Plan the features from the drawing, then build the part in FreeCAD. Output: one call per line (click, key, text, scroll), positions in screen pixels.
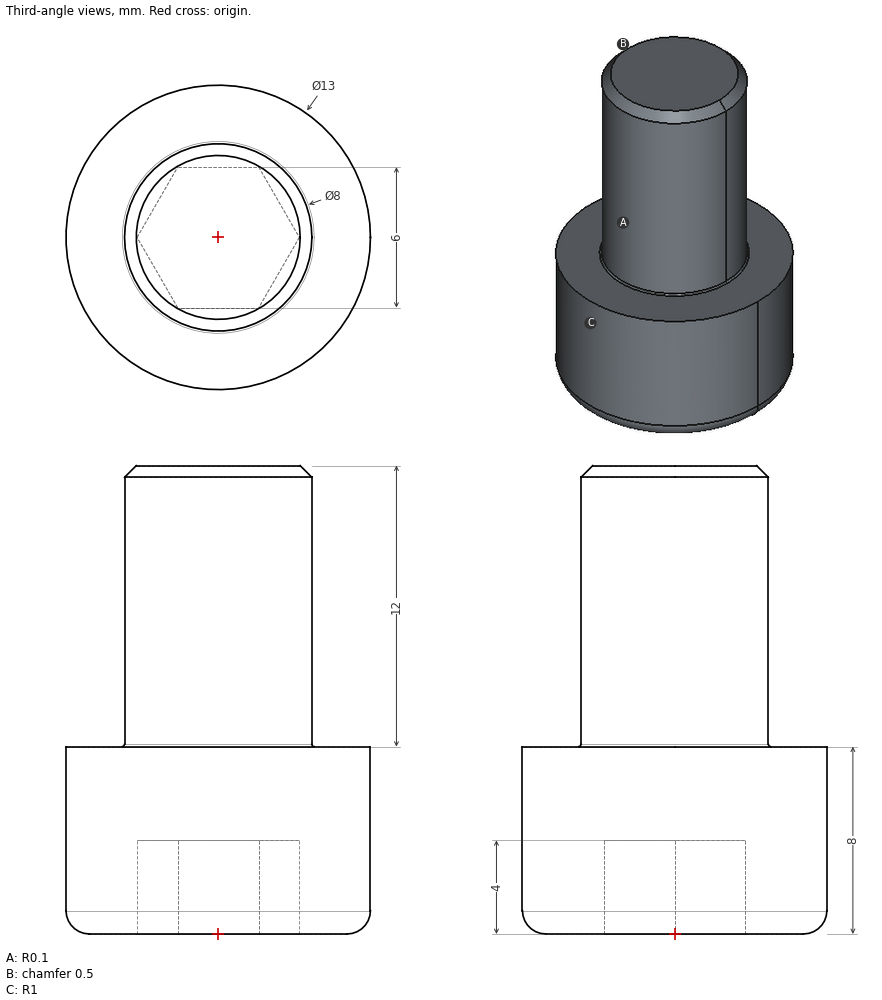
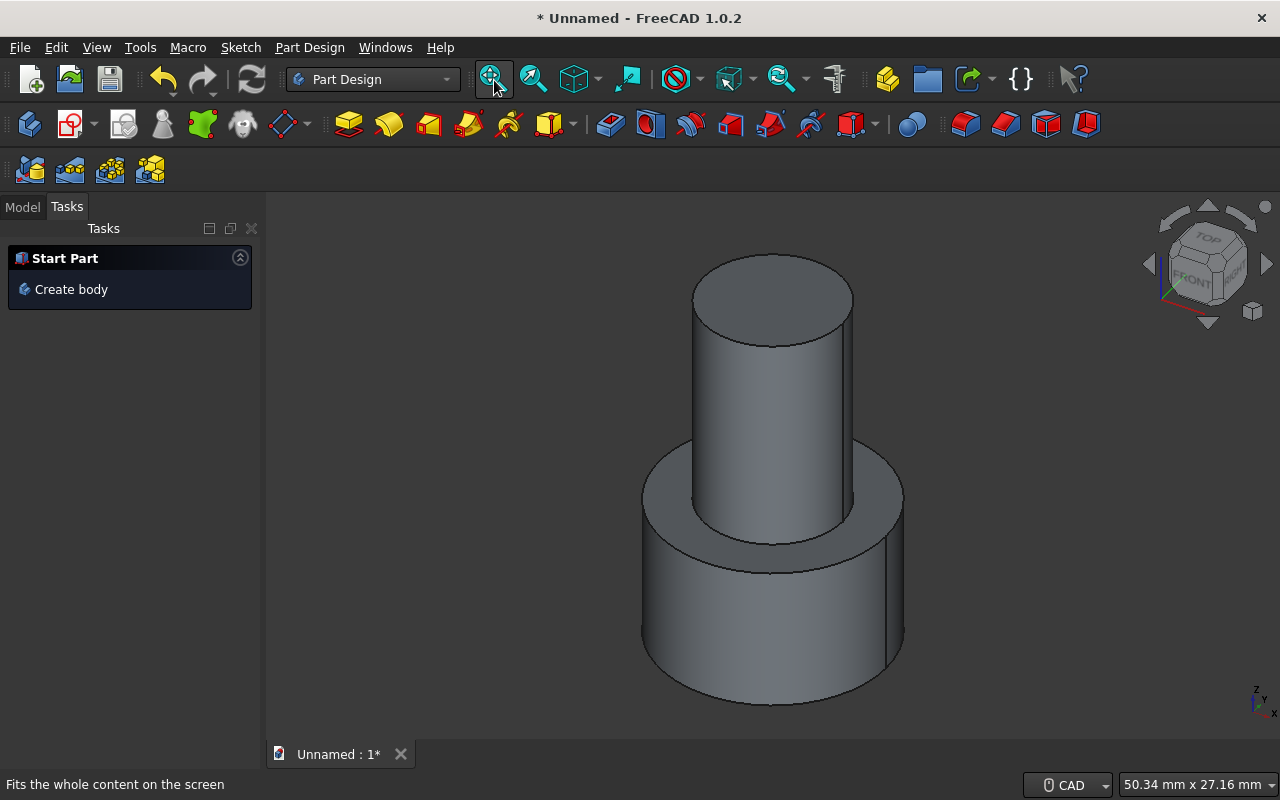
click(70, 124)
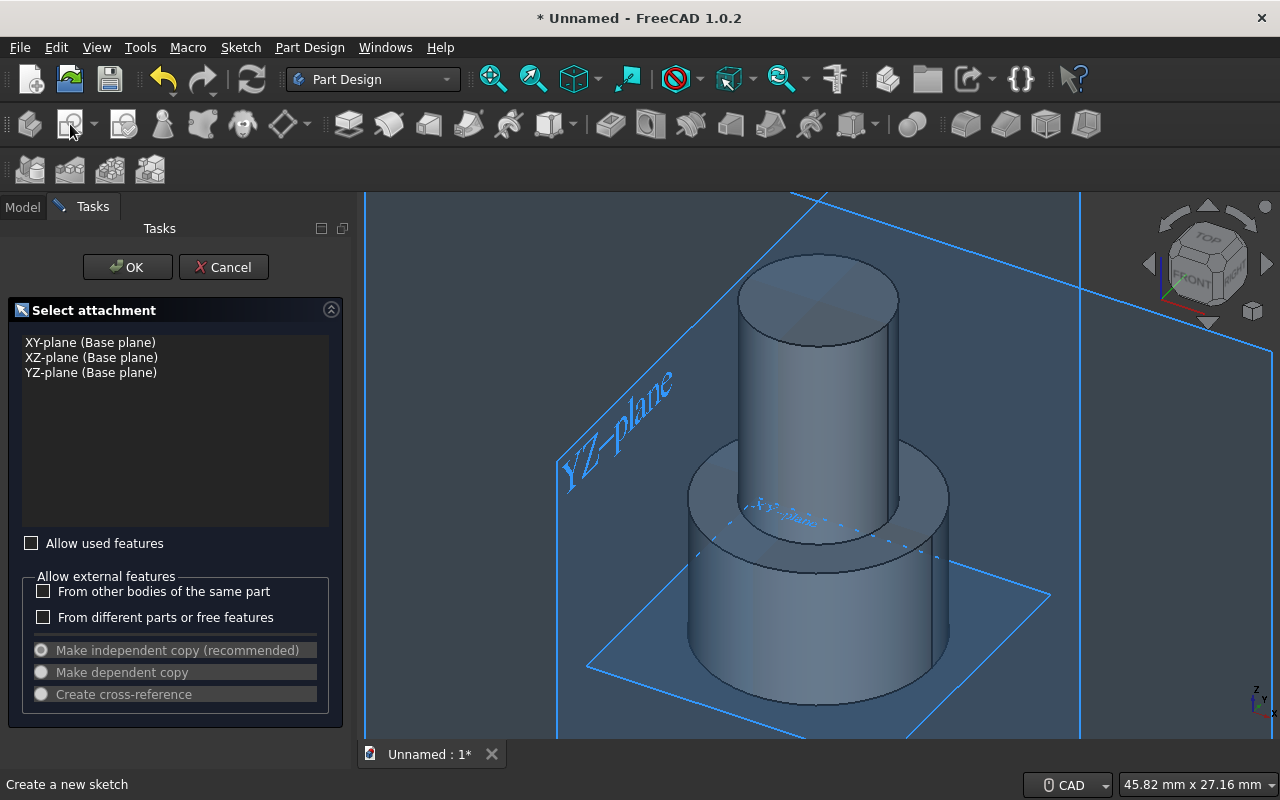
click(82, 342)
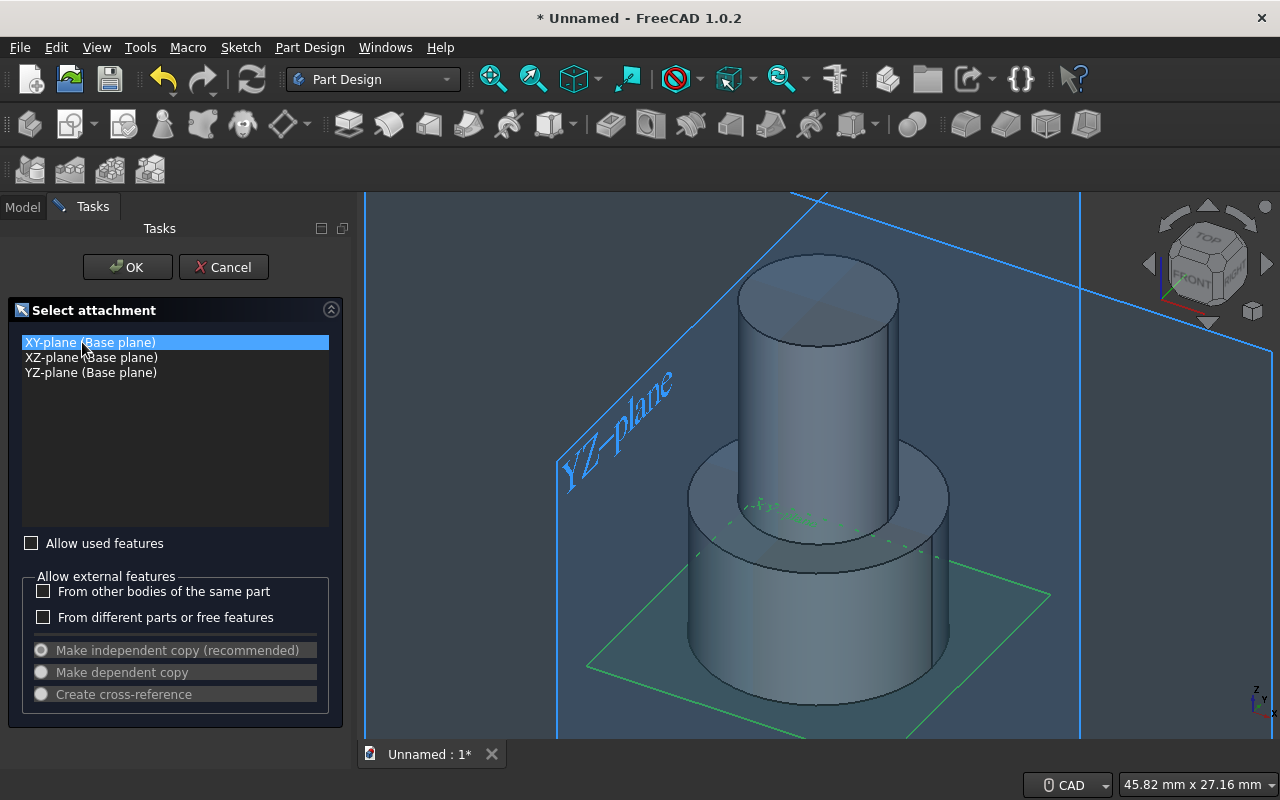
click(128, 267)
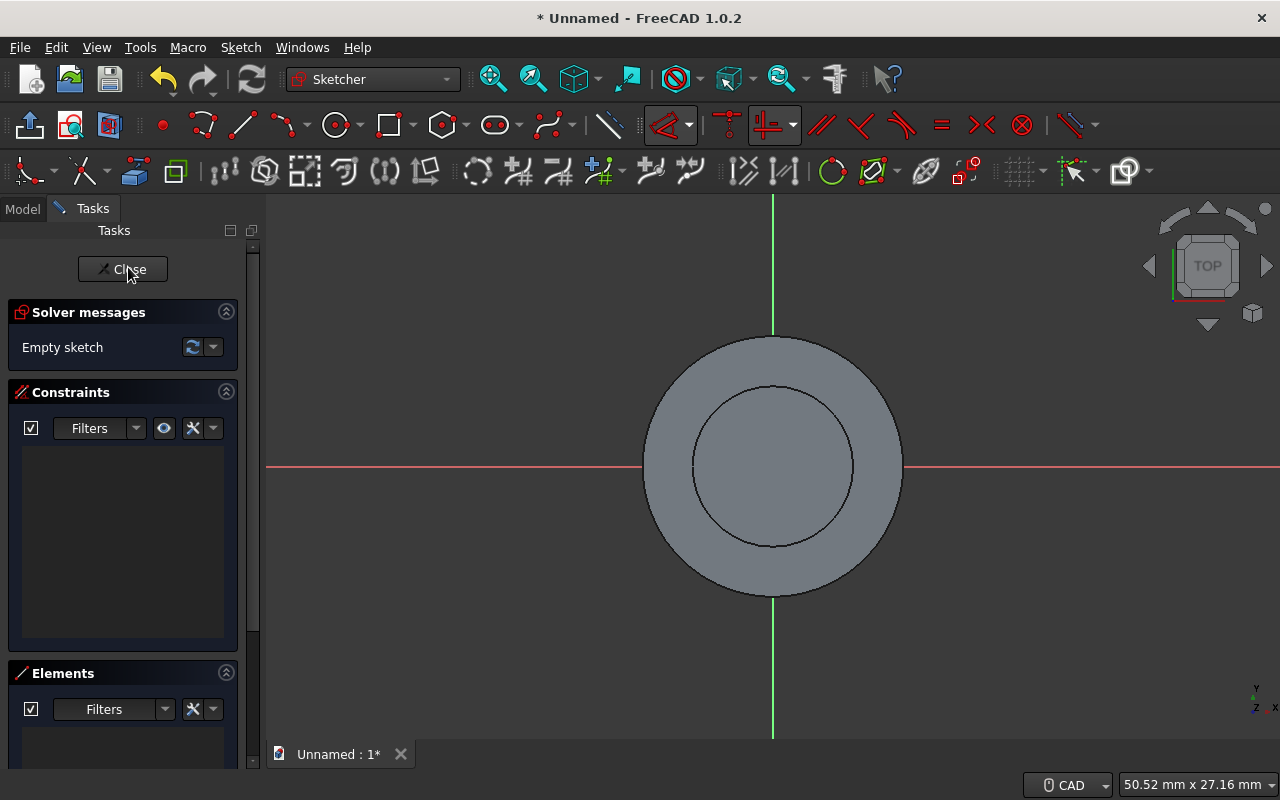
click(110, 126)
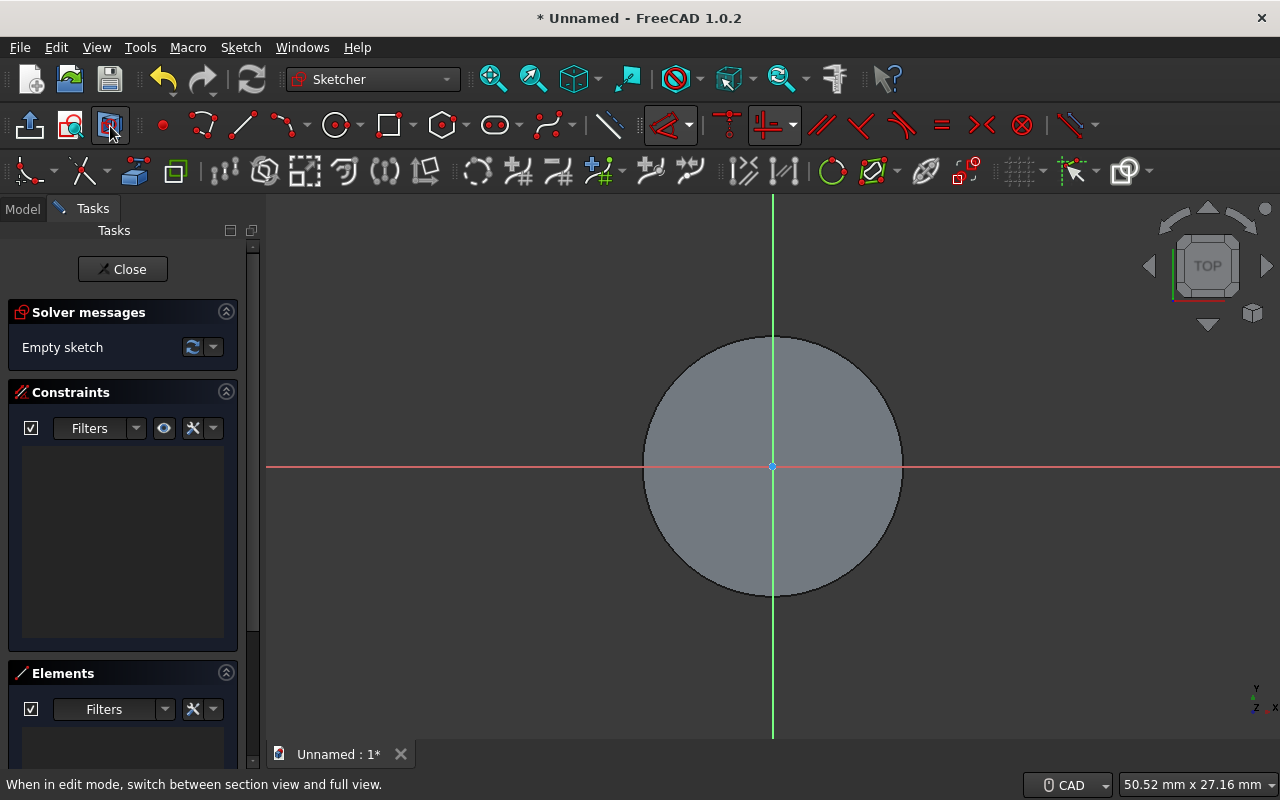
scroll(813, 466, up, 5)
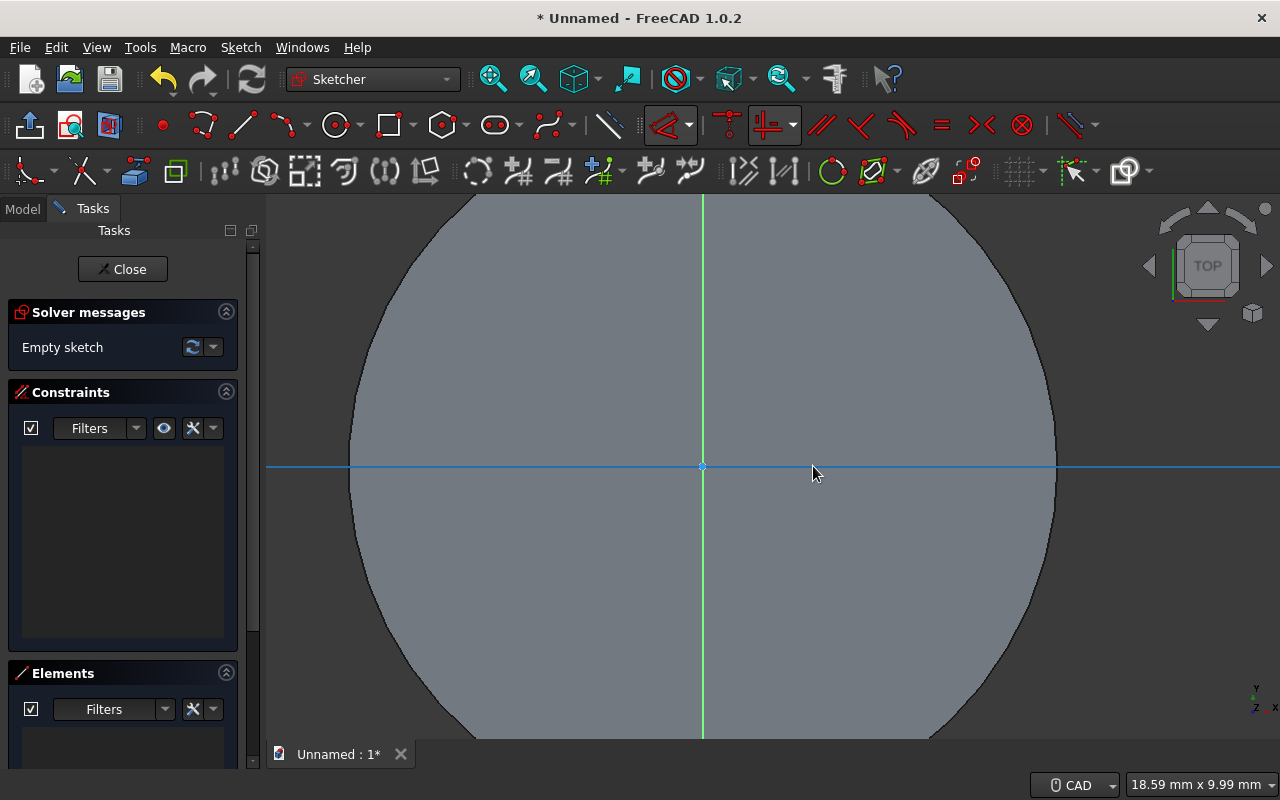
click(442, 126)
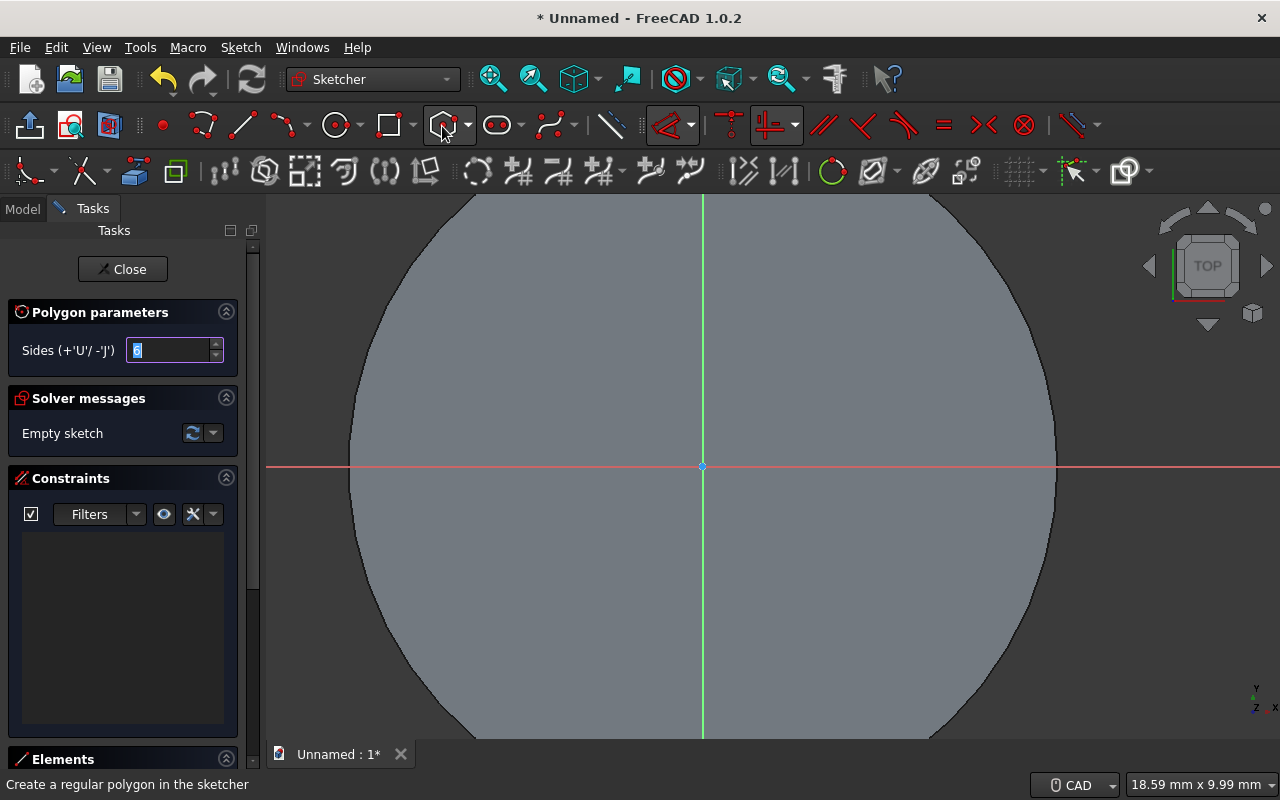
click(703, 466)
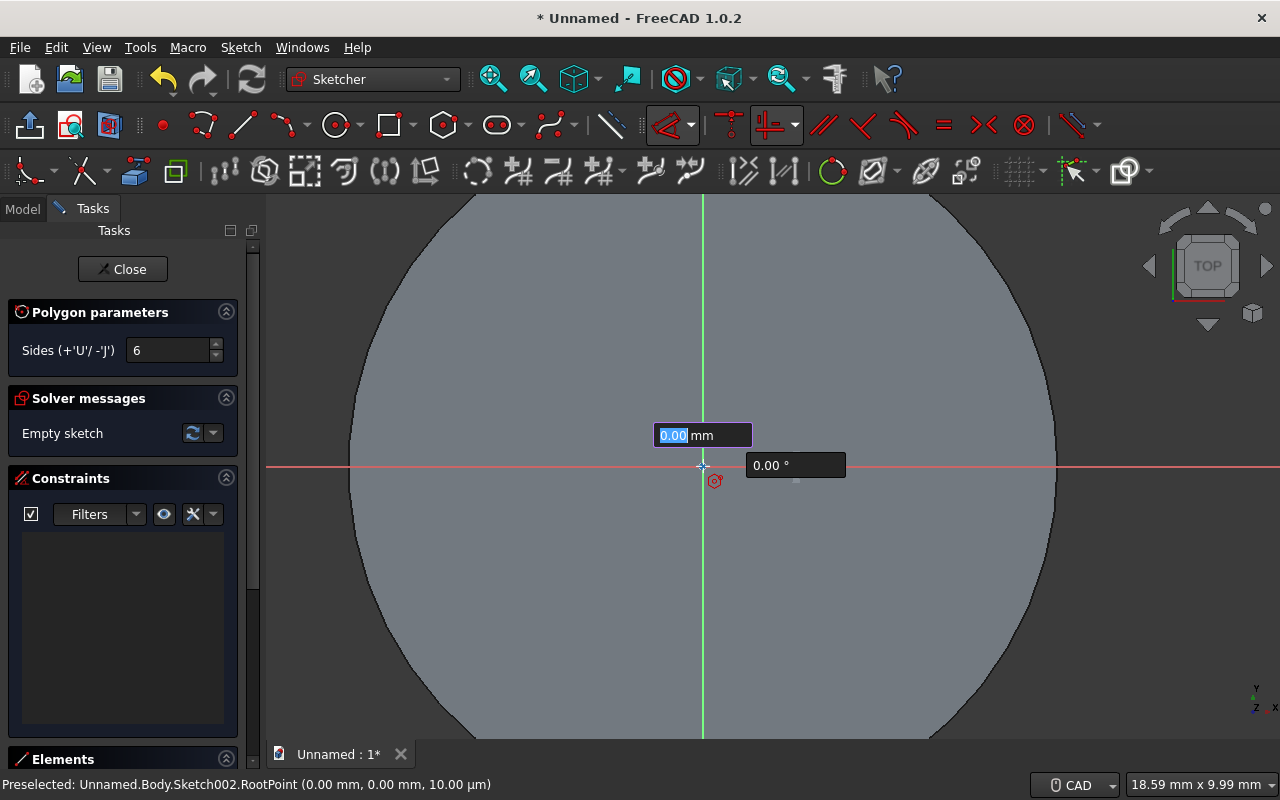
click(514, 466)
right_click(514, 466)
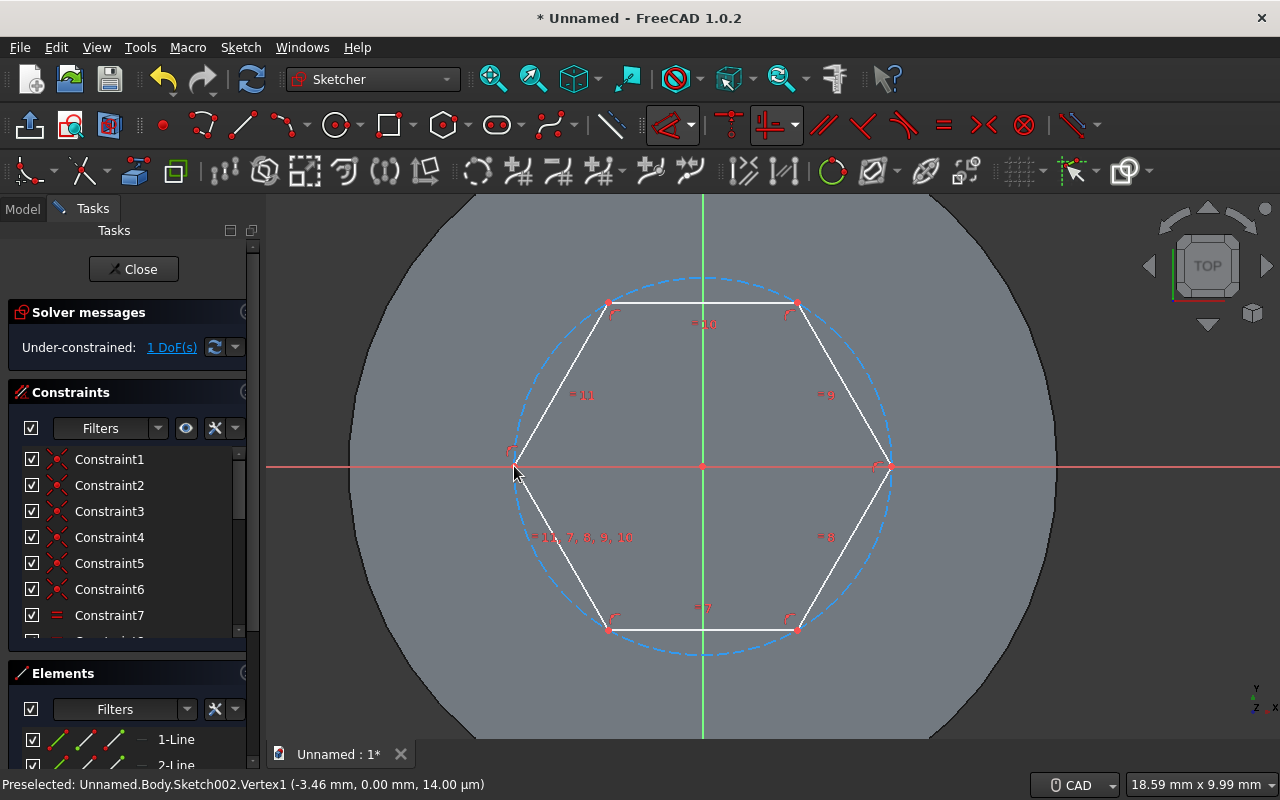
click(608, 630)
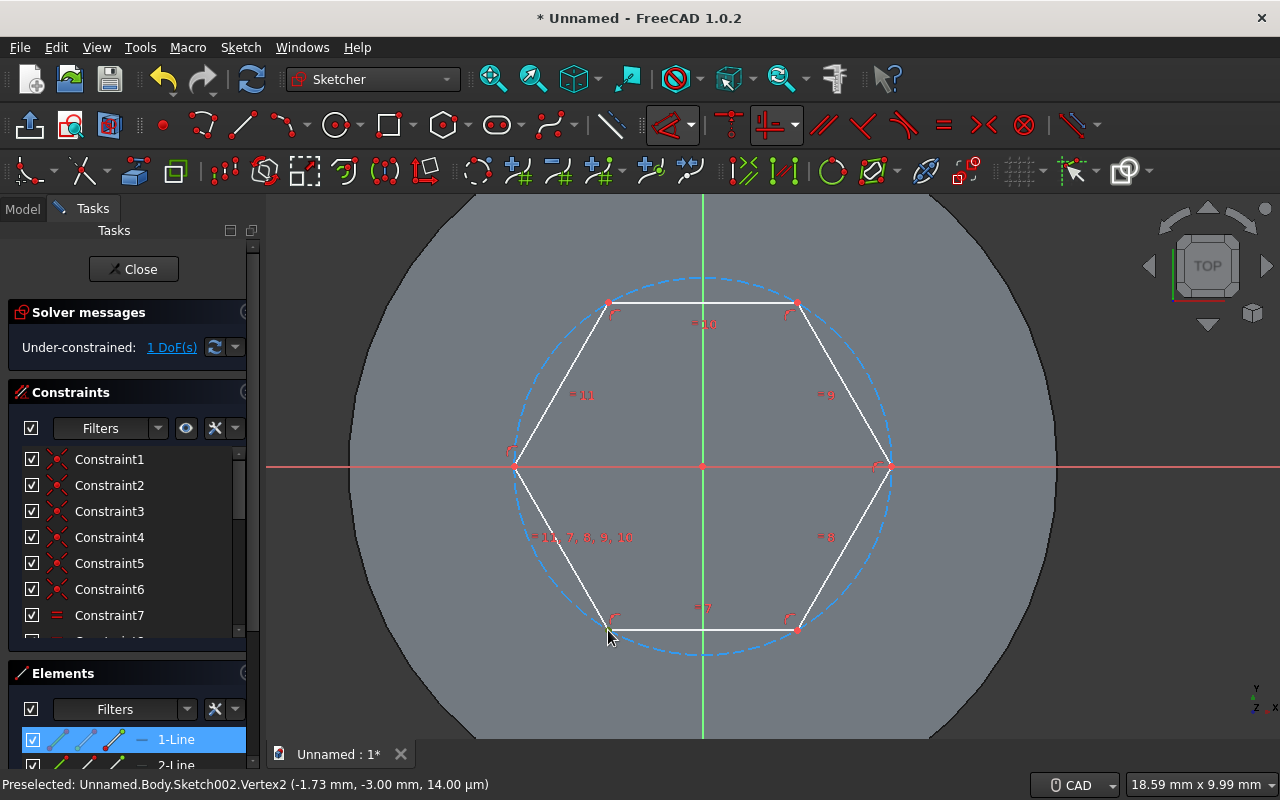
click(797, 303)